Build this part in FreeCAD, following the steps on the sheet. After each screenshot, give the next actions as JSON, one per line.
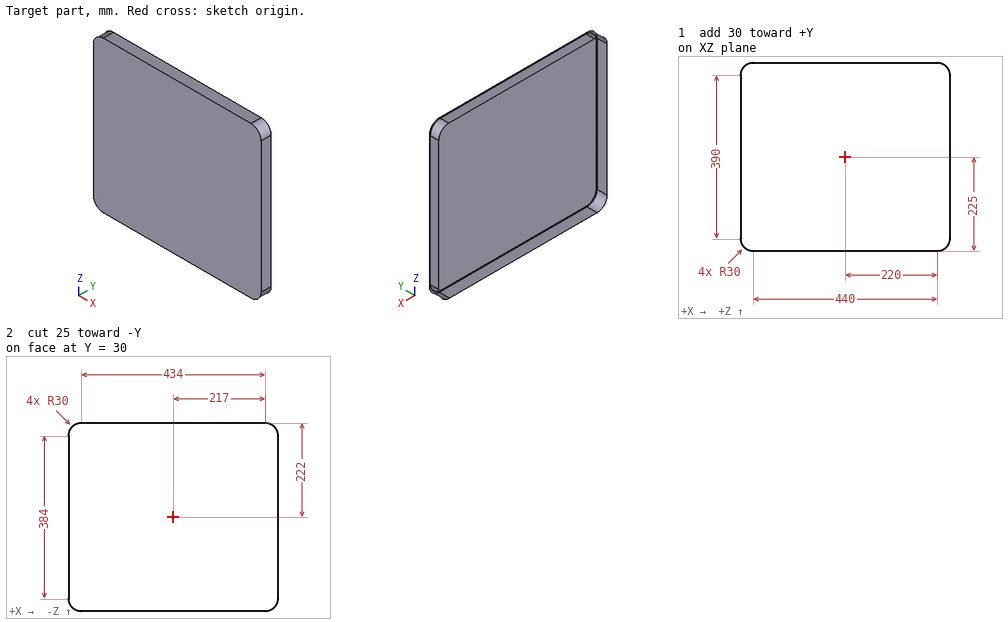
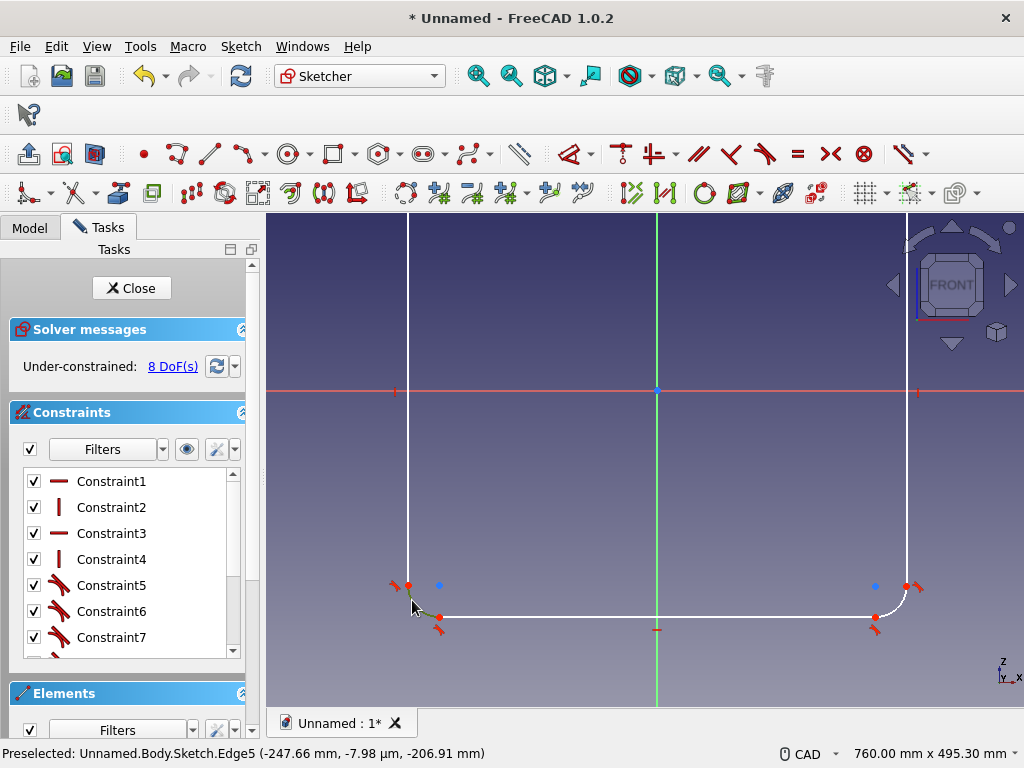
{"action": "scroll", "coordinate": [412, 600], "scroll_direction": "down", "scroll_amount": 2}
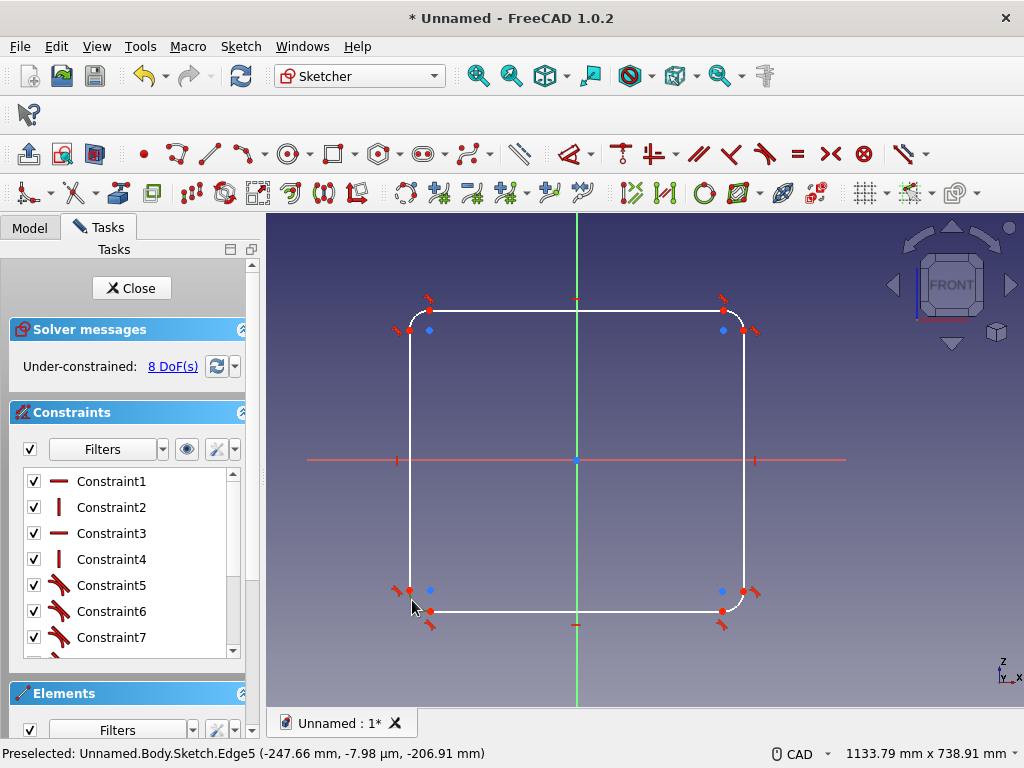
{"action": "scroll", "coordinate": [420, 313], "scroll_direction": "up", "scroll_amount": 2}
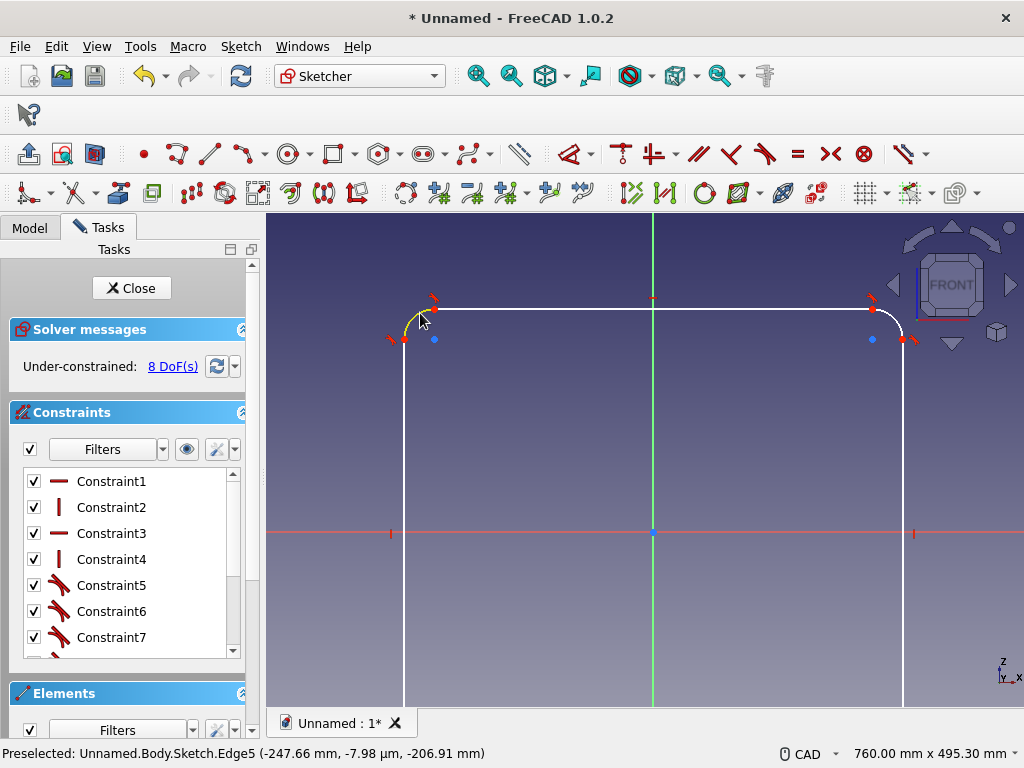
{"action": "left_click", "coordinate": [421, 313]}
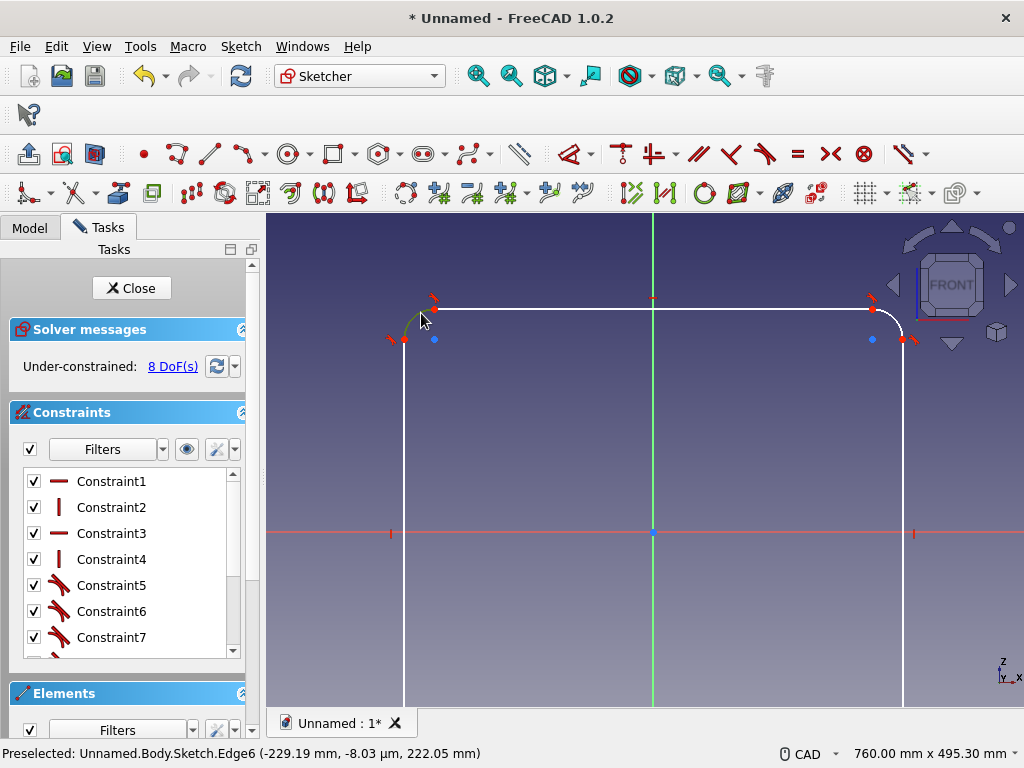
{"action": "scroll", "coordinate": [420, 313], "scroll_direction": "down", "scroll_amount": 2}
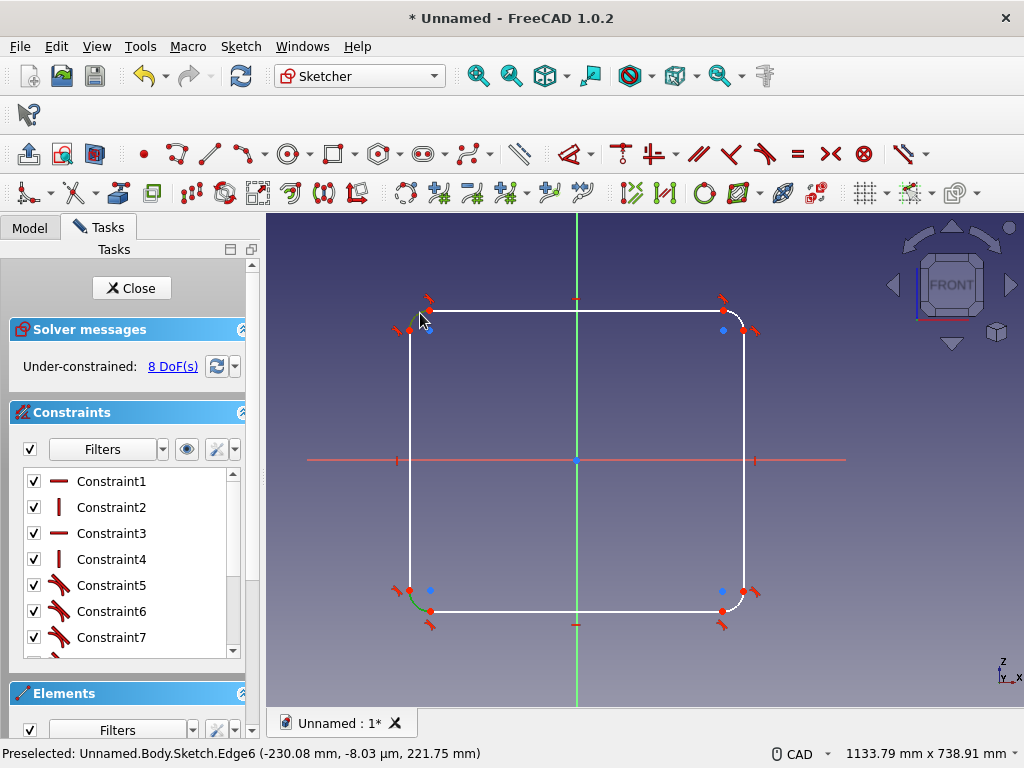
{"action": "scroll", "coordinate": [741, 322], "scroll_direction": "up", "scroll_amount": 2}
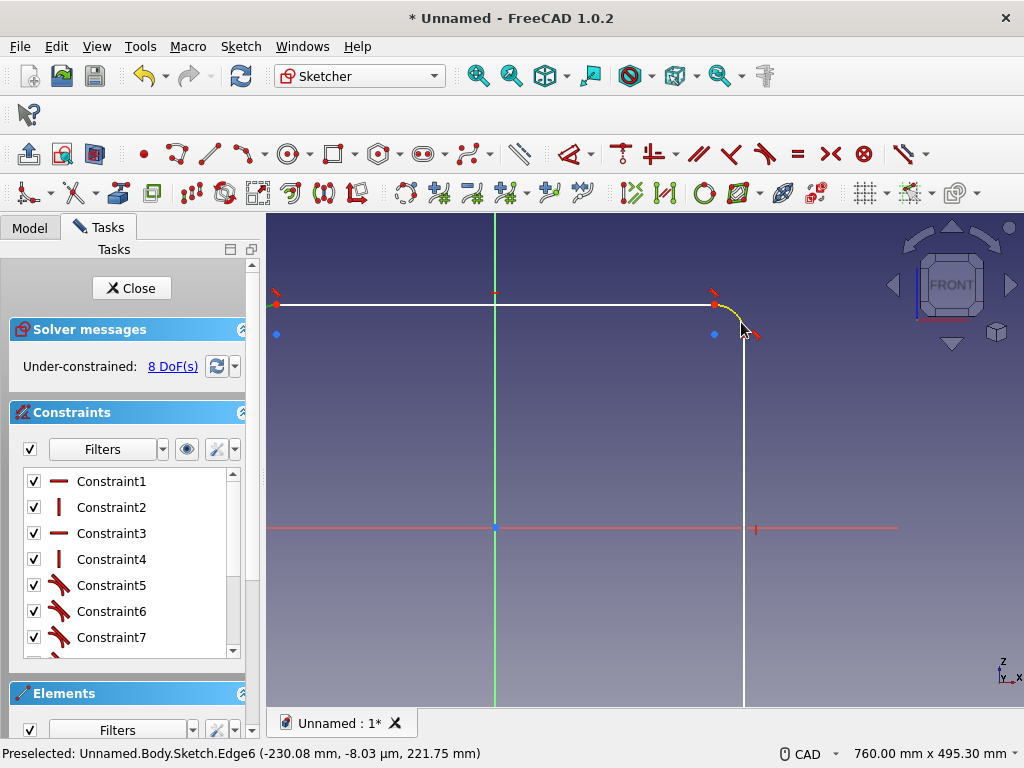
{"action": "left_click", "coordinate": [741, 321]}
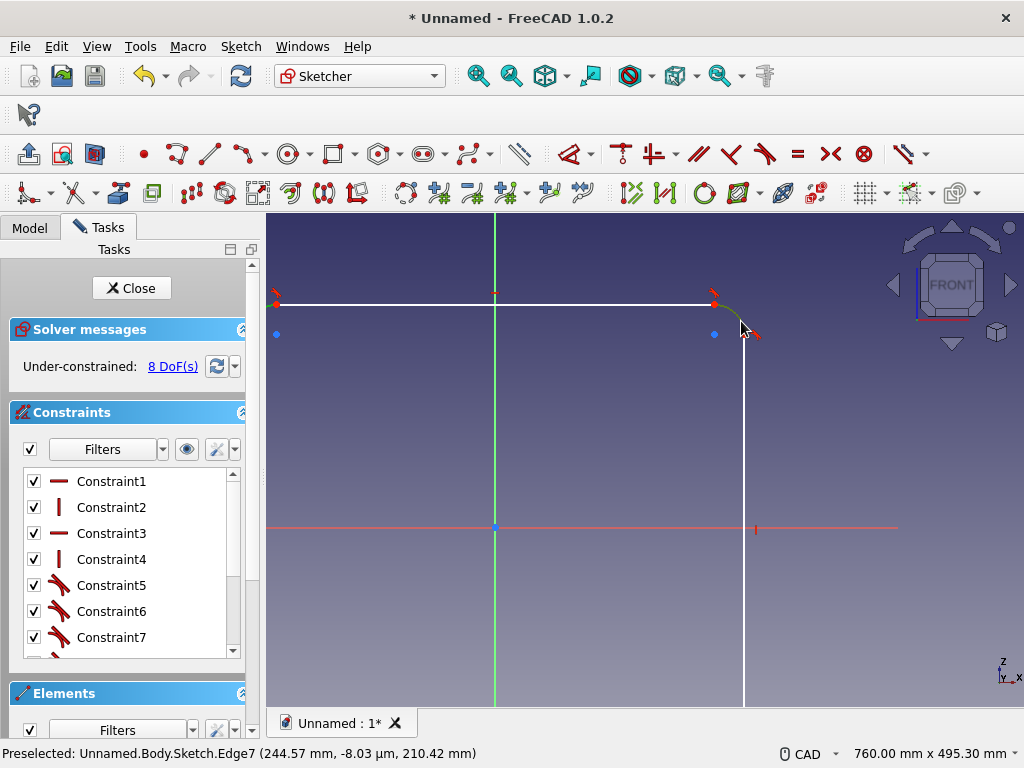
{"action": "scroll", "coordinate": [741, 322], "scroll_direction": "down", "scroll_amount": 2}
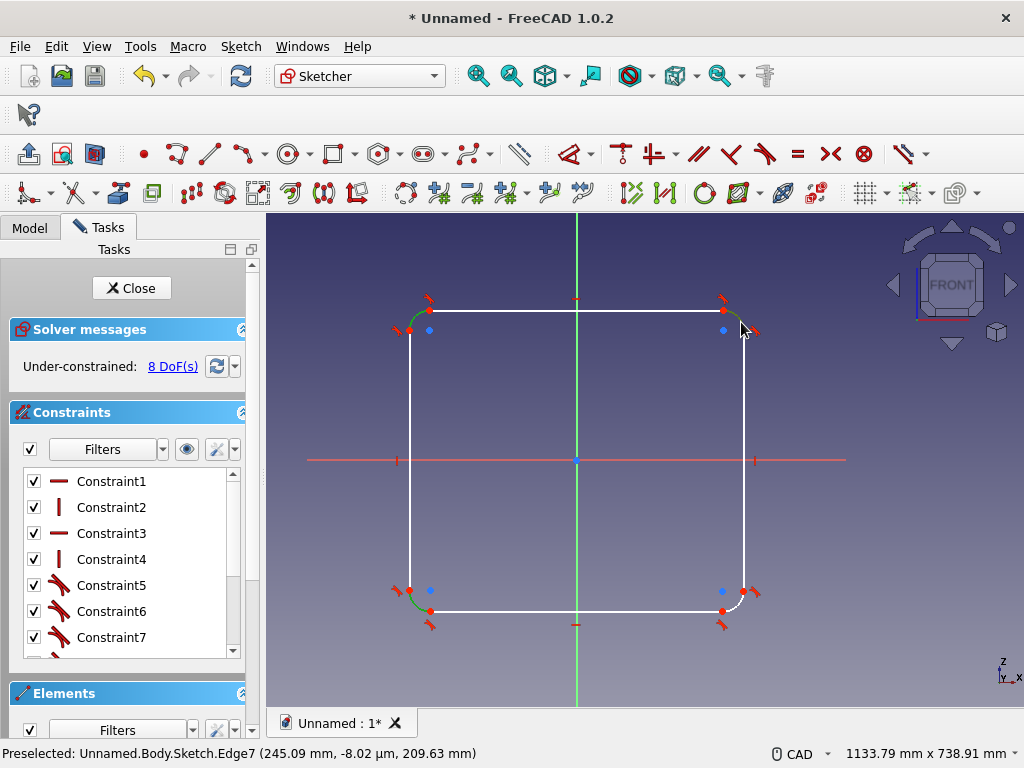
{"action": "scroll", "coordinate": [732, 609], "scroll_direction": "up", "scroll_amount": 2}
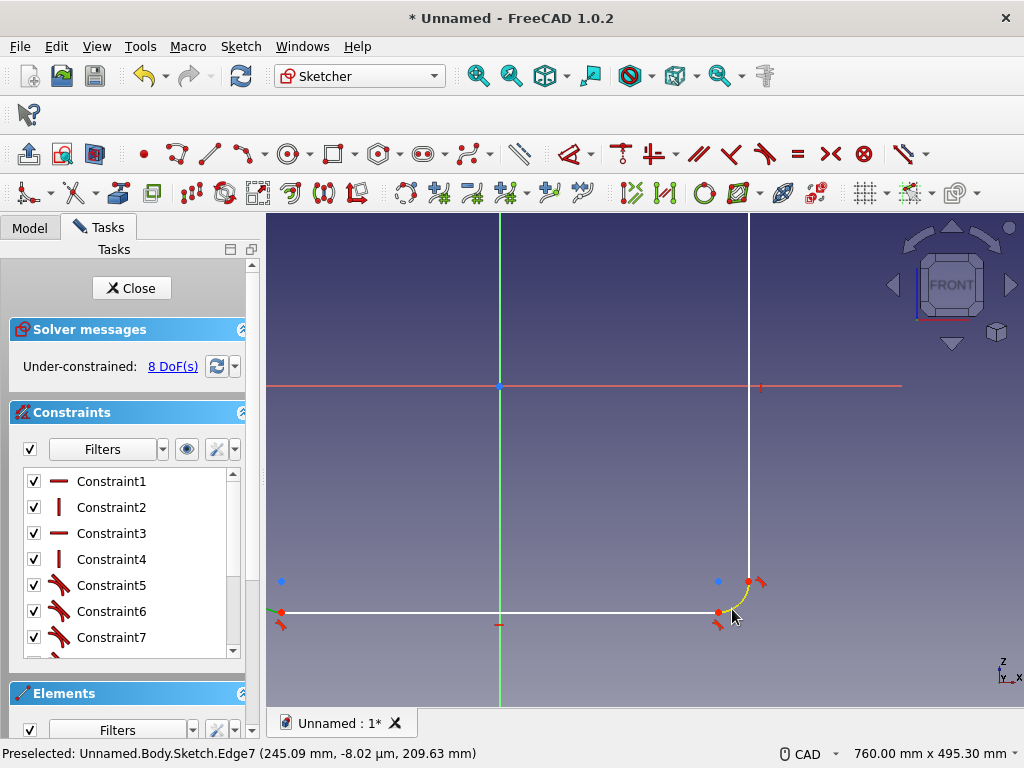
{"action": "left_click", "coordinate": [732, 609]}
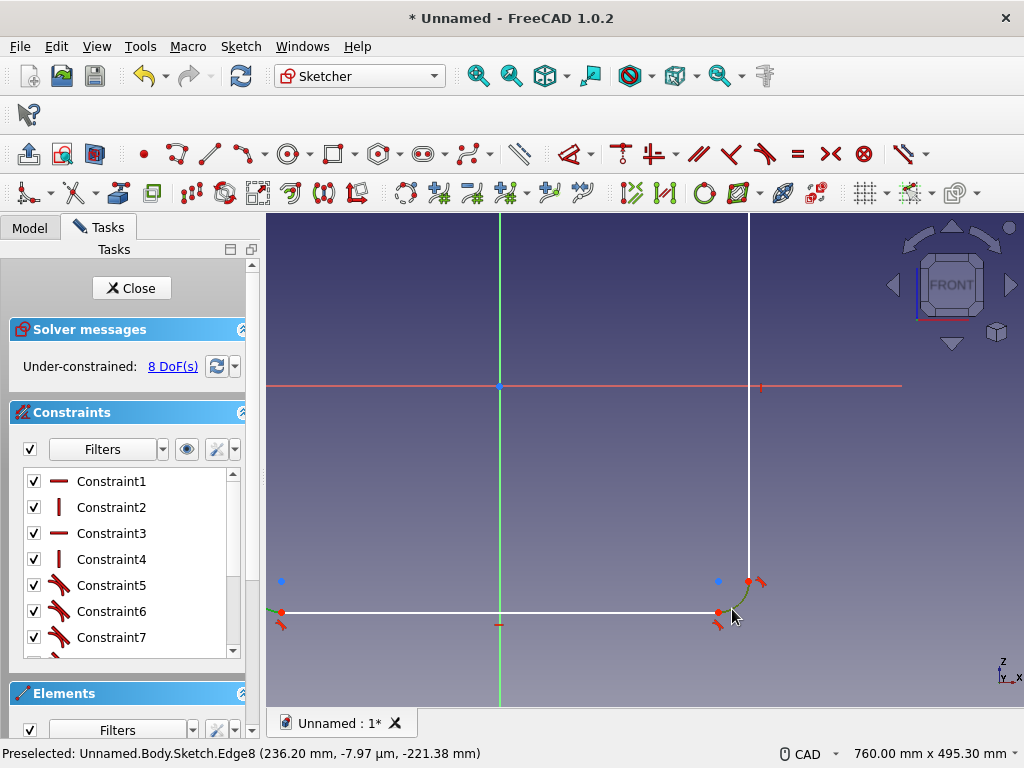
{"action": "left_click", "coordinate": [798, 154]}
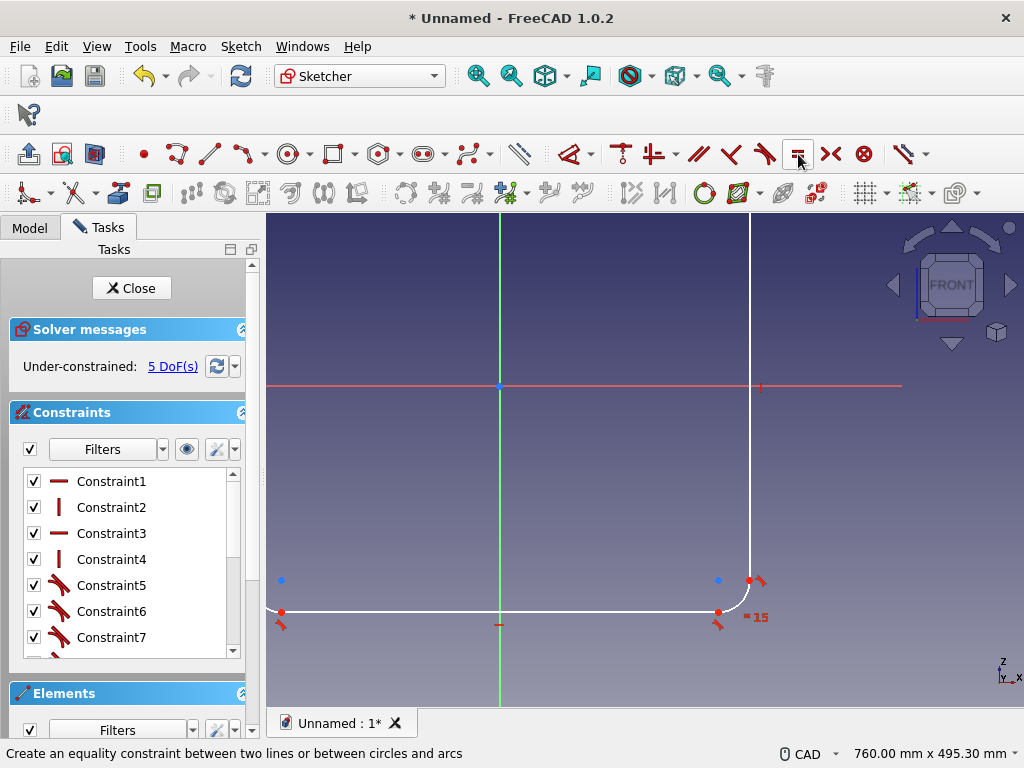
{"action": "left_click", "coordinate": [568, 154]}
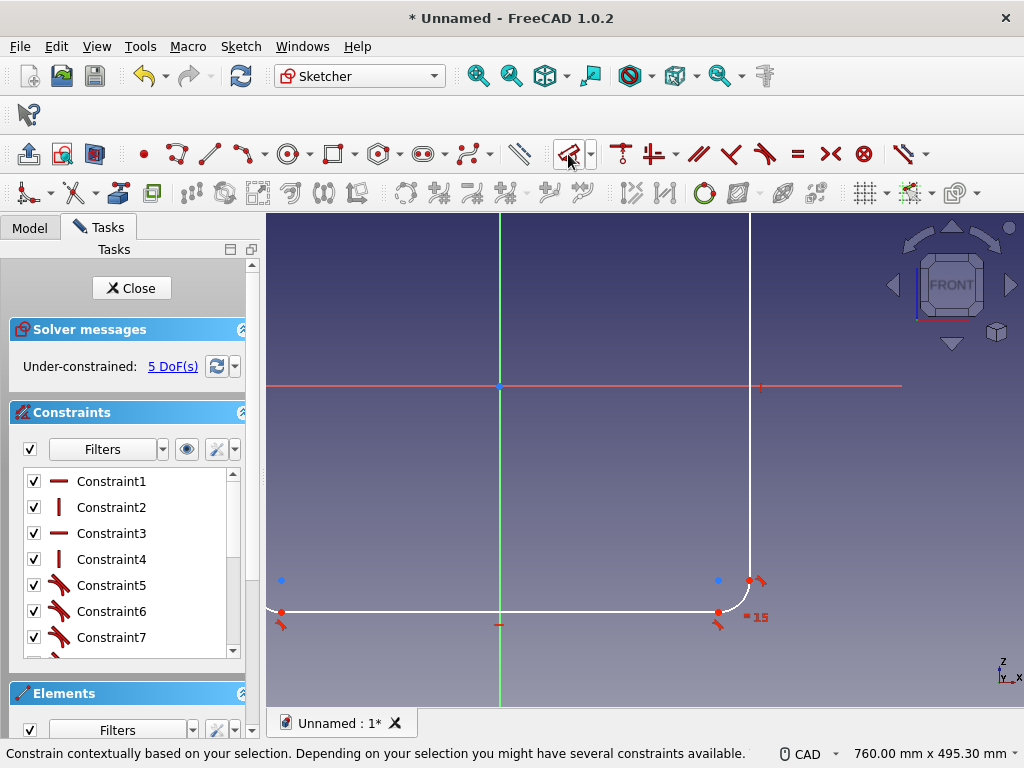
{"action": "scroll", "coordinate": [732, 609], "scroll_direction": "down", "scroll_amount": 2}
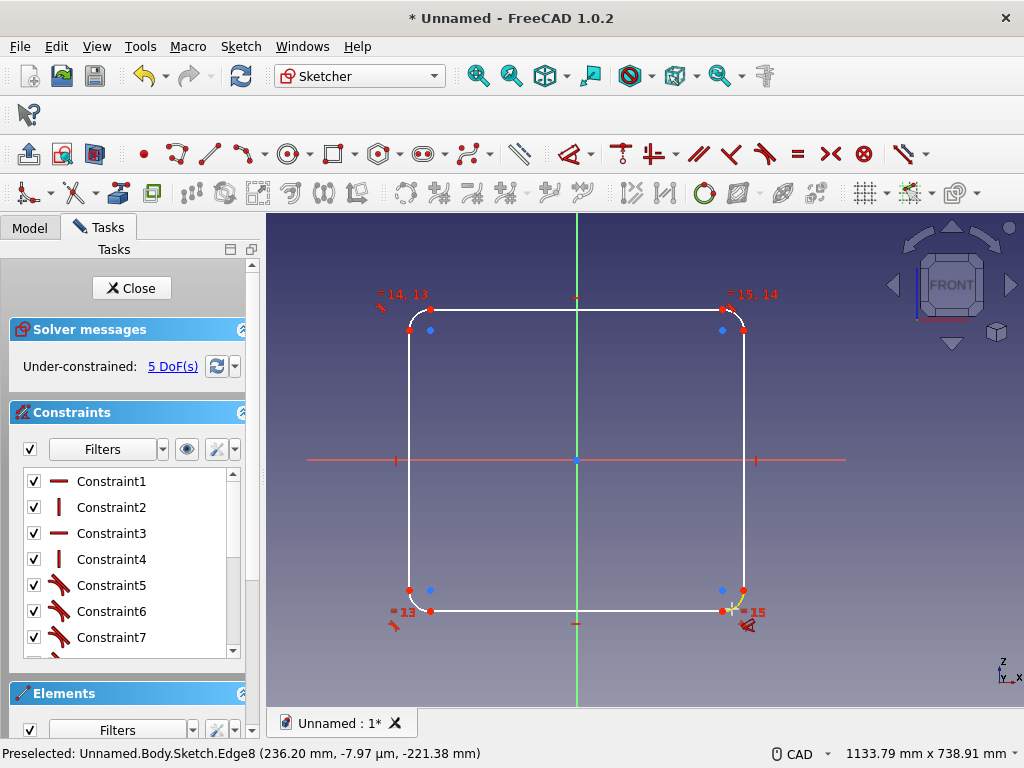
{"action": "scroll", "coordinate": [412, 600], "scroll_direction": "up", "scroll_amount": 4}